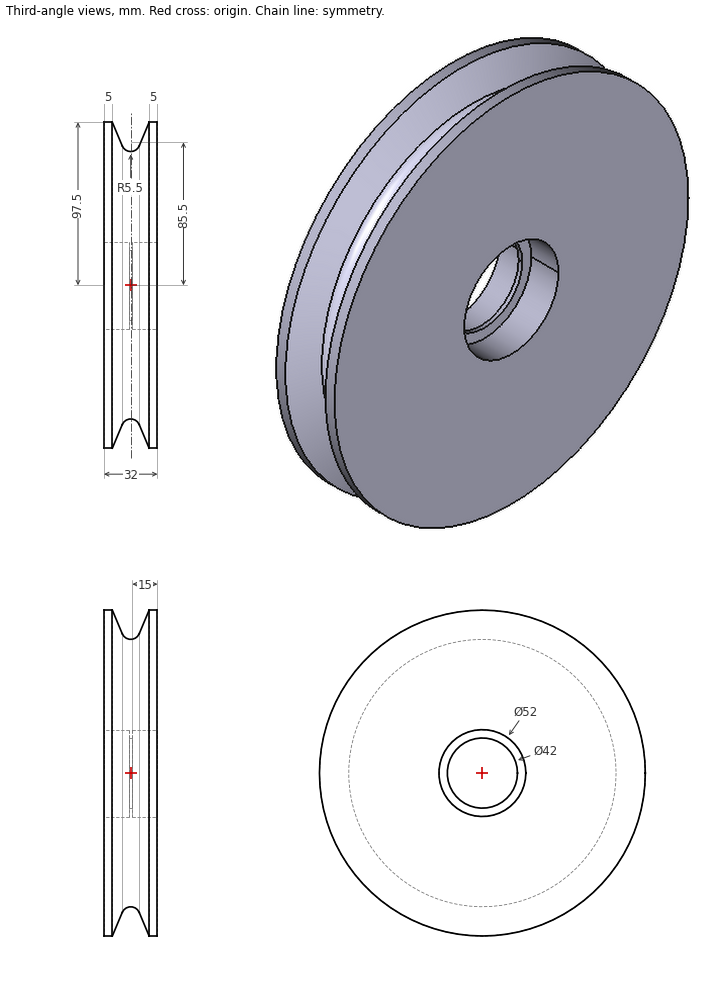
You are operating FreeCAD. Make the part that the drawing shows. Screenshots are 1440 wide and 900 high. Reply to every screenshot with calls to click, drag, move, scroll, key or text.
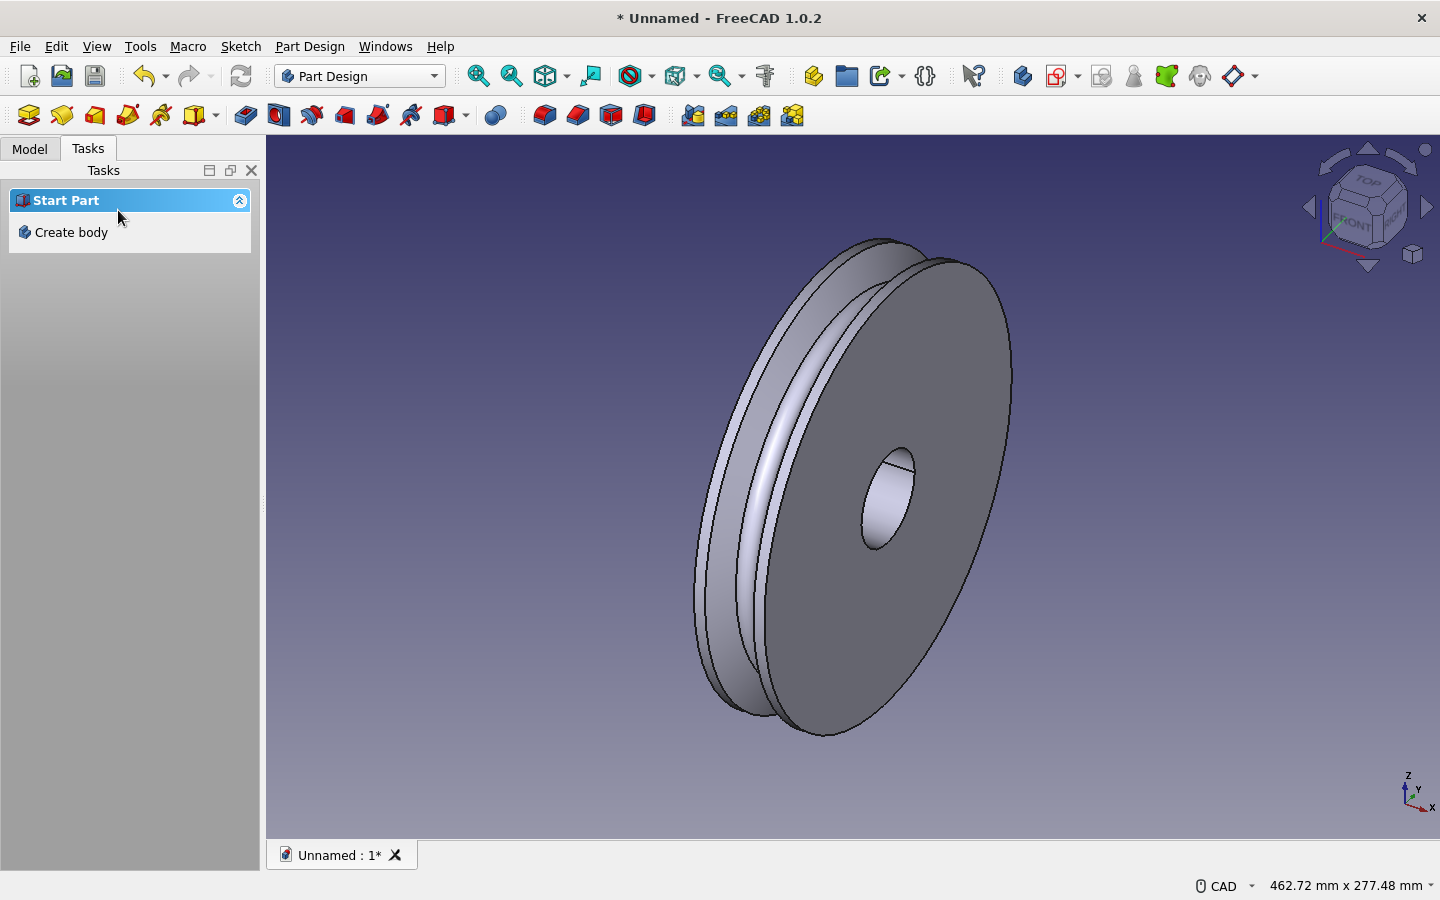
click(959, 485)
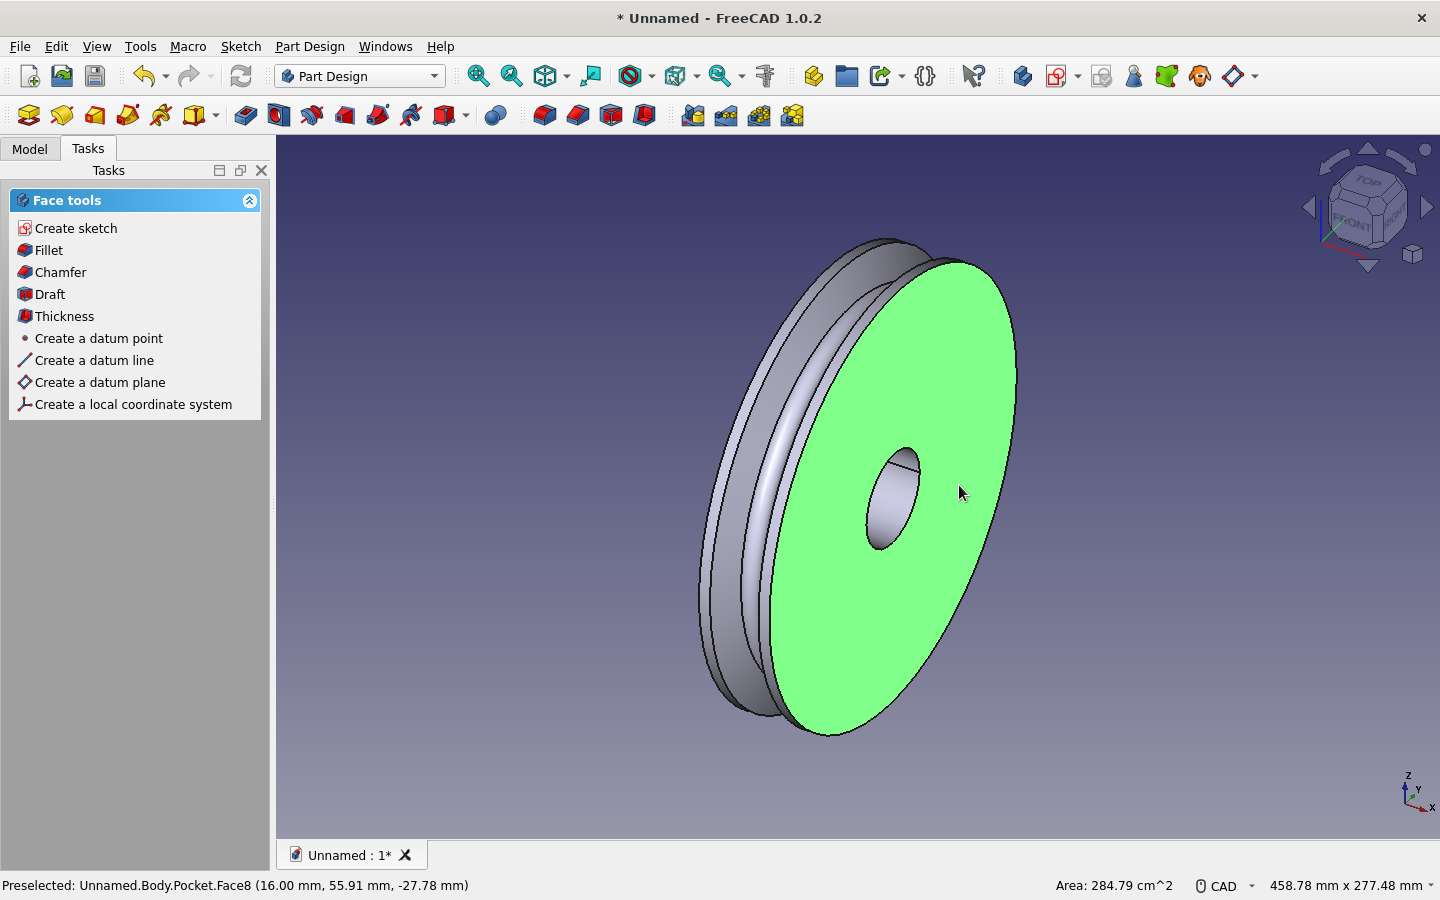
click(1056, 76)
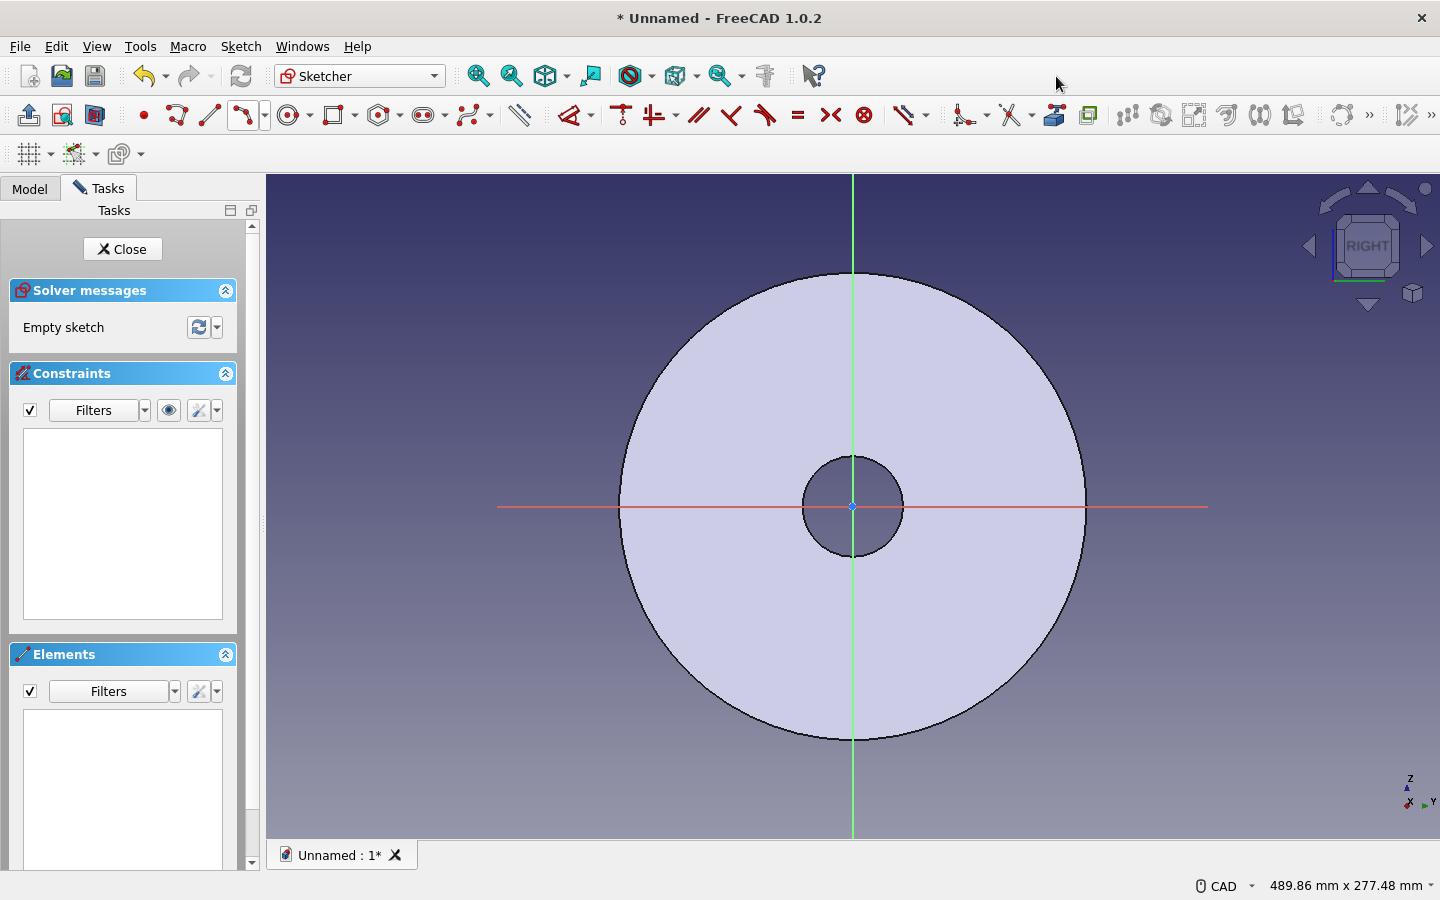
scroll(882, 506, up, 6)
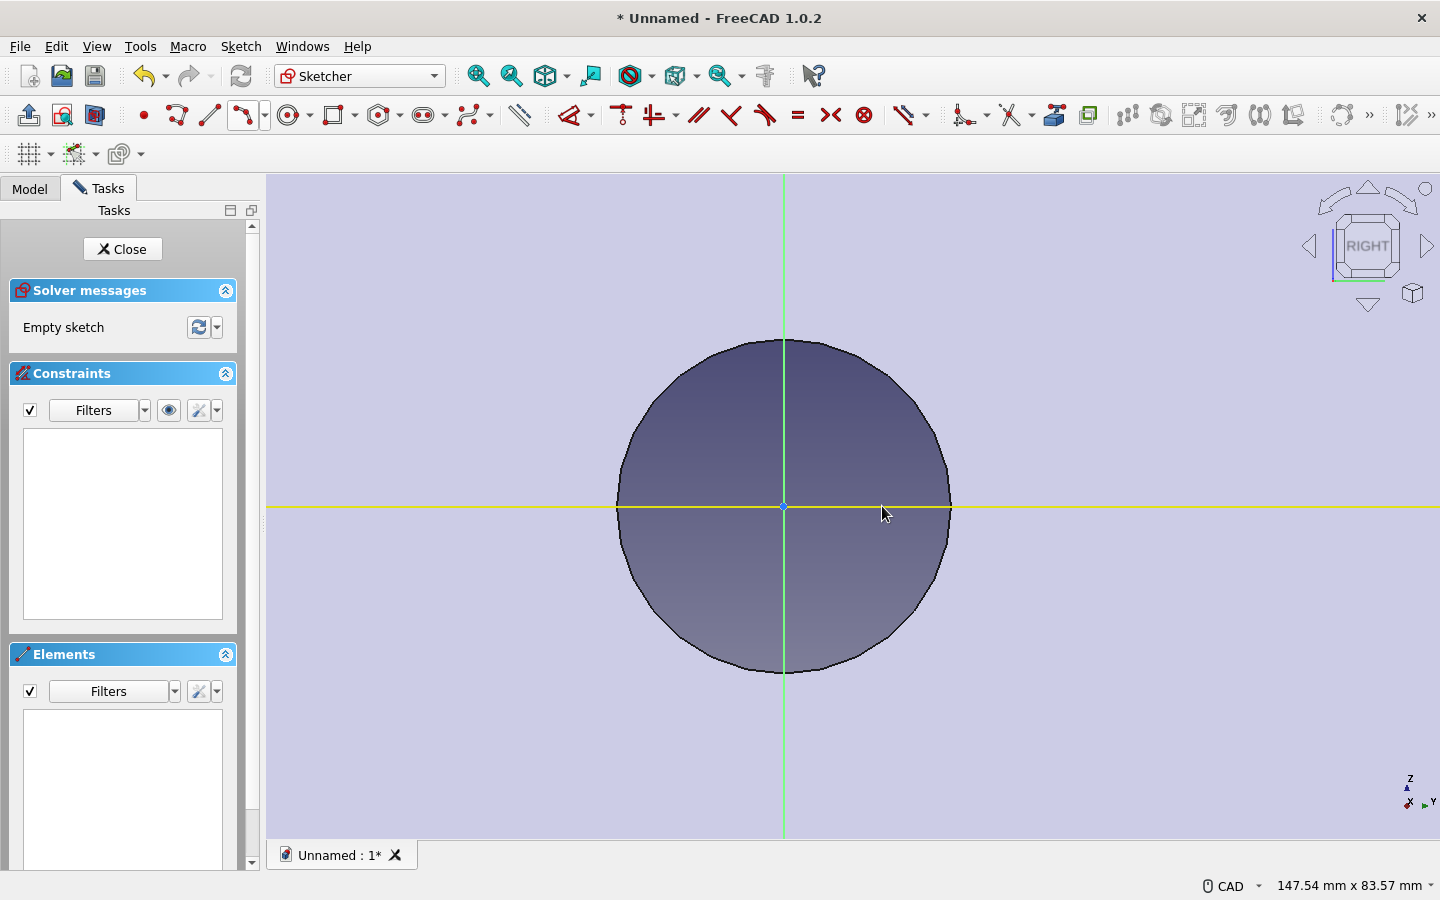
click(288, 116)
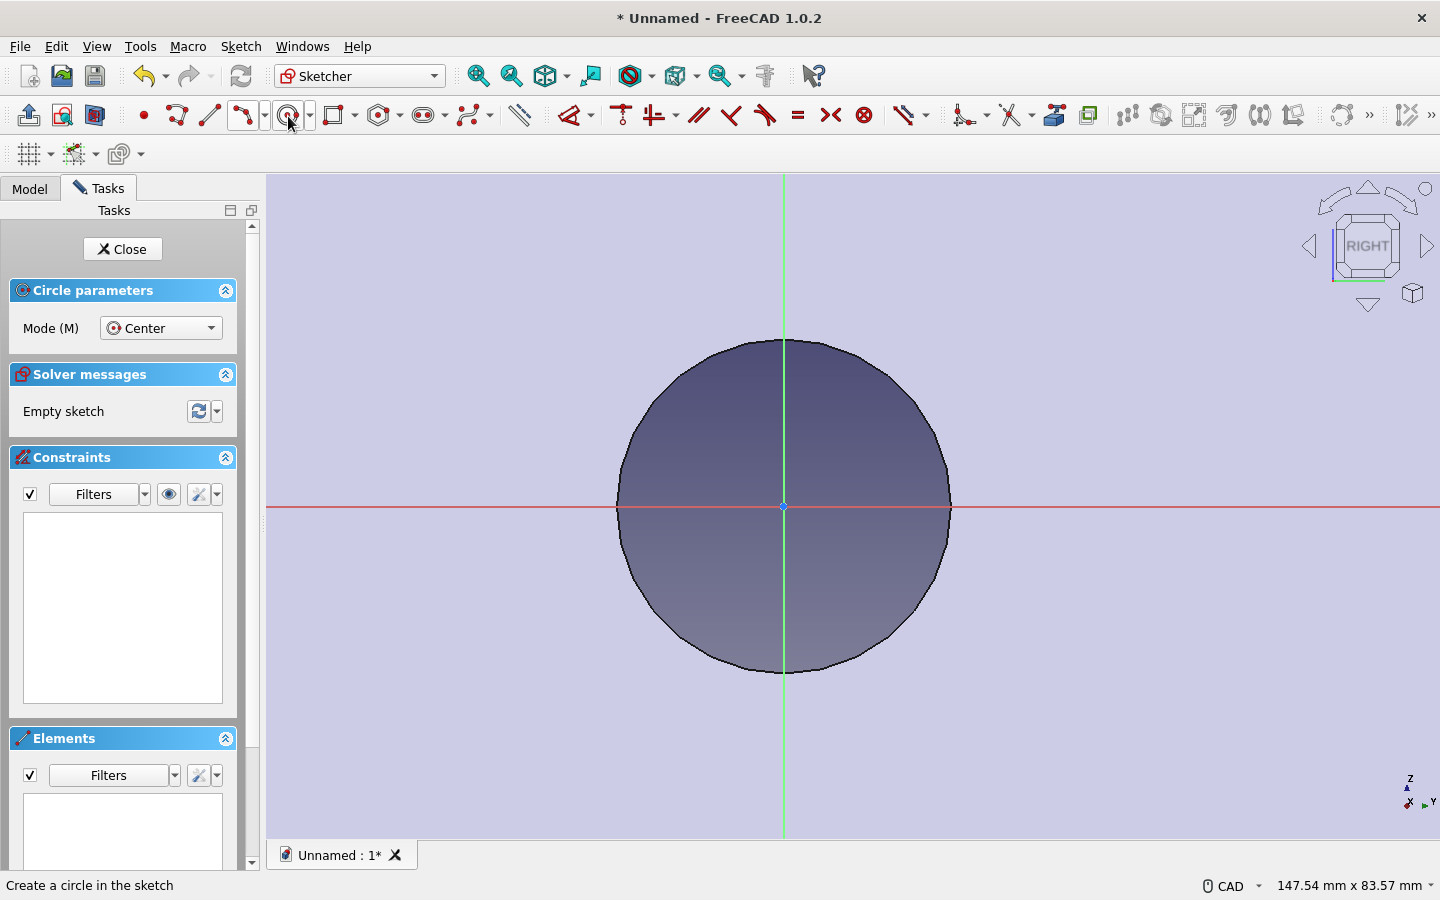
click(784, 506)
click(930, 360)
key(Escape)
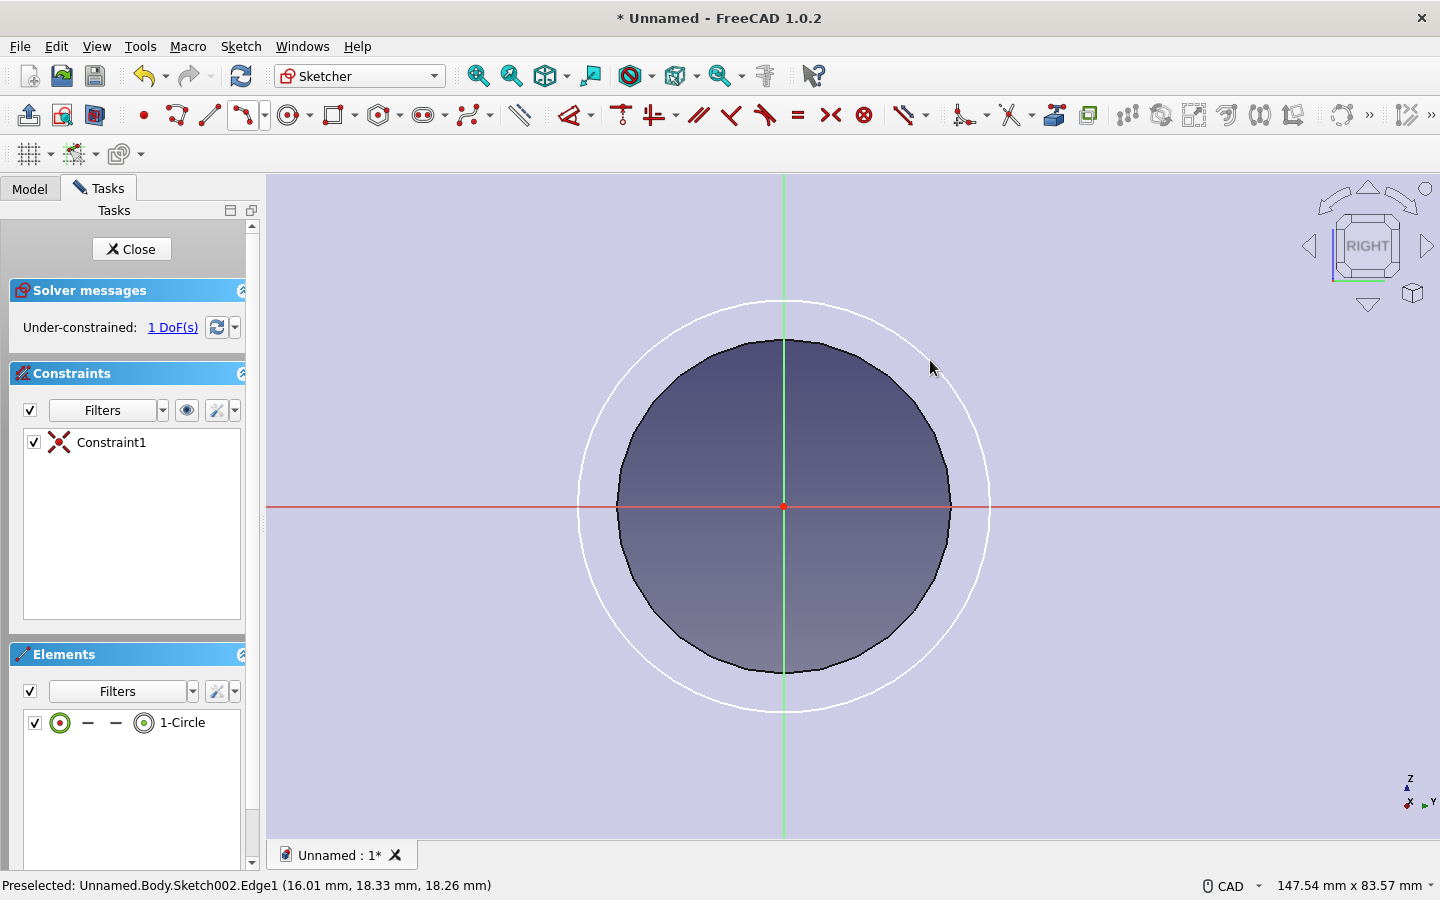
click(568, 116)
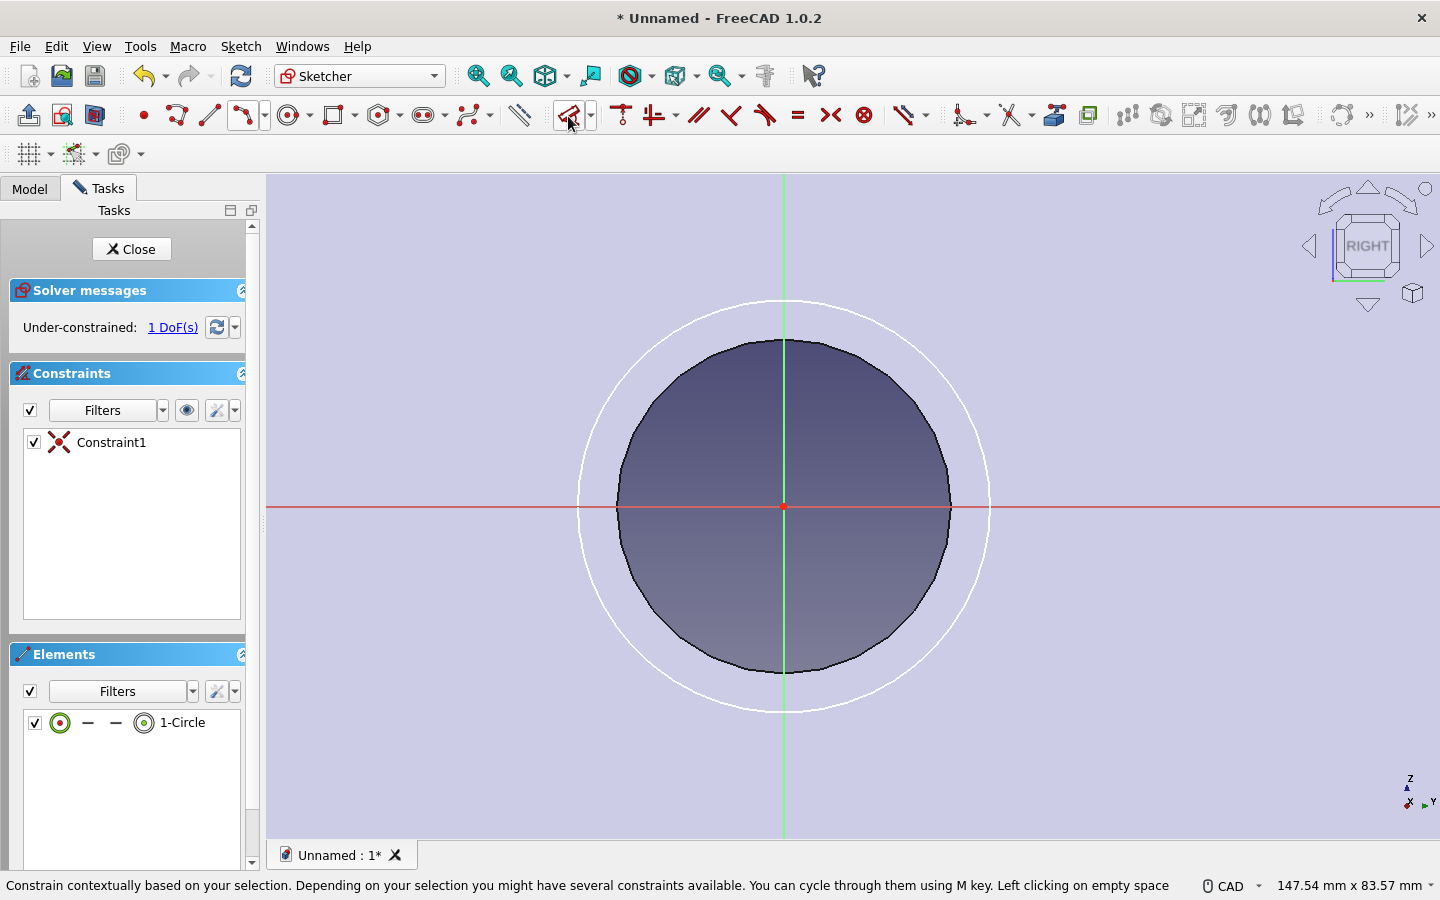
click(929, 360)
click(952, 337)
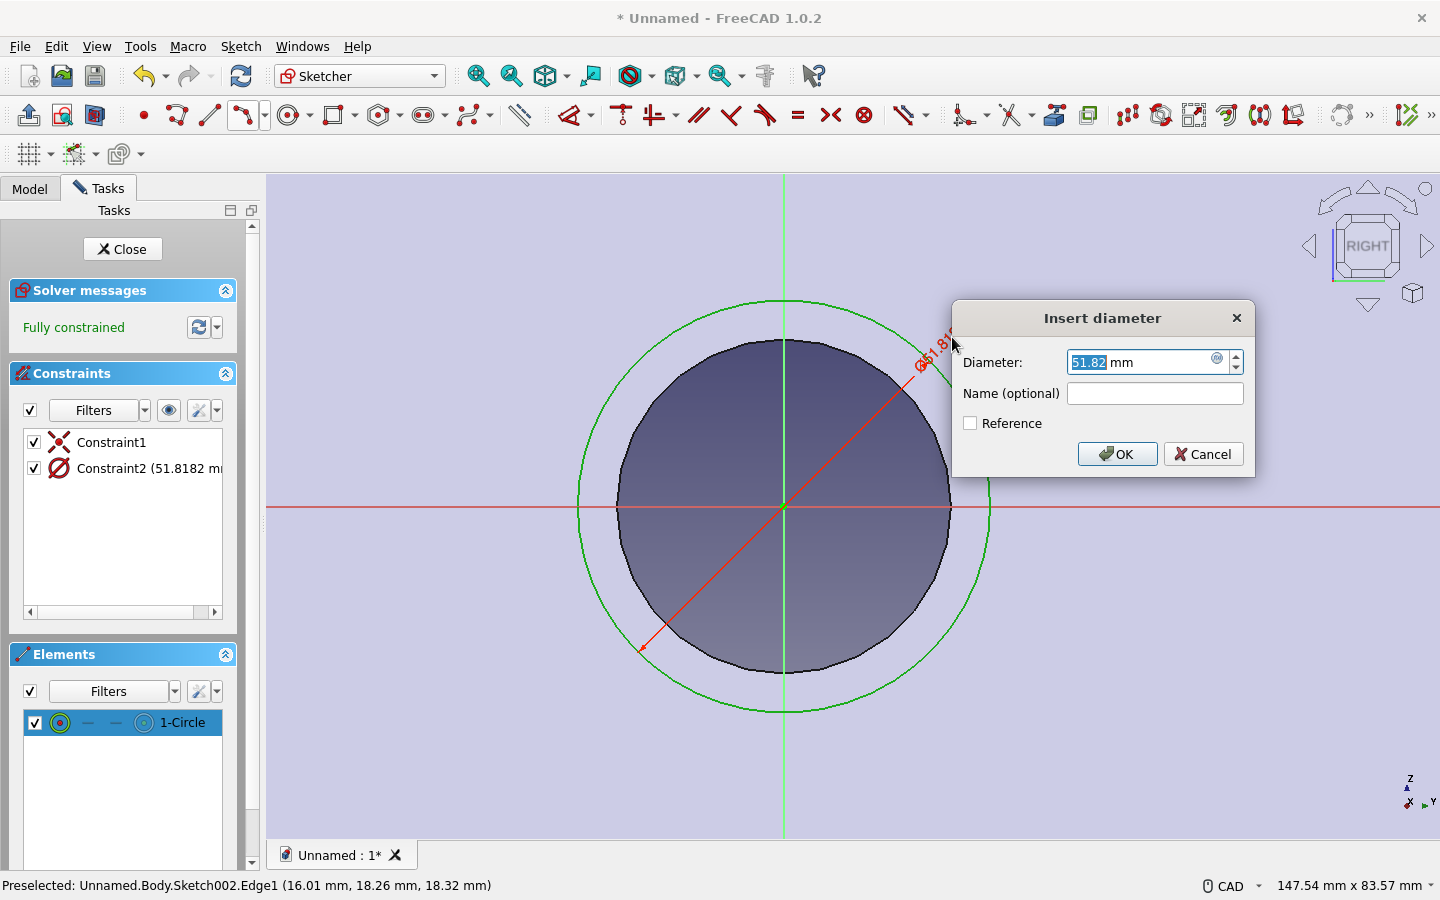
text(52)
key(Return)
key(Escape)